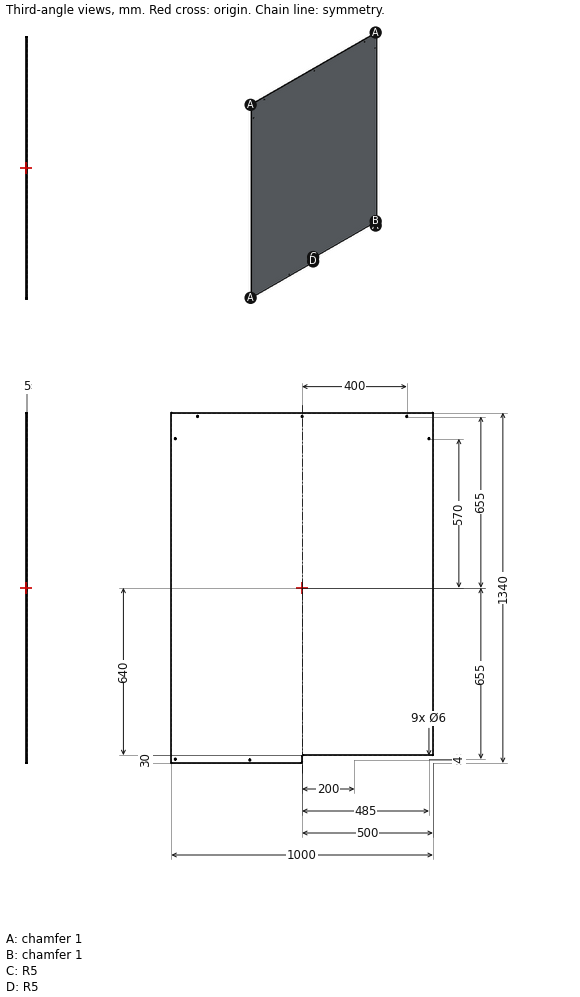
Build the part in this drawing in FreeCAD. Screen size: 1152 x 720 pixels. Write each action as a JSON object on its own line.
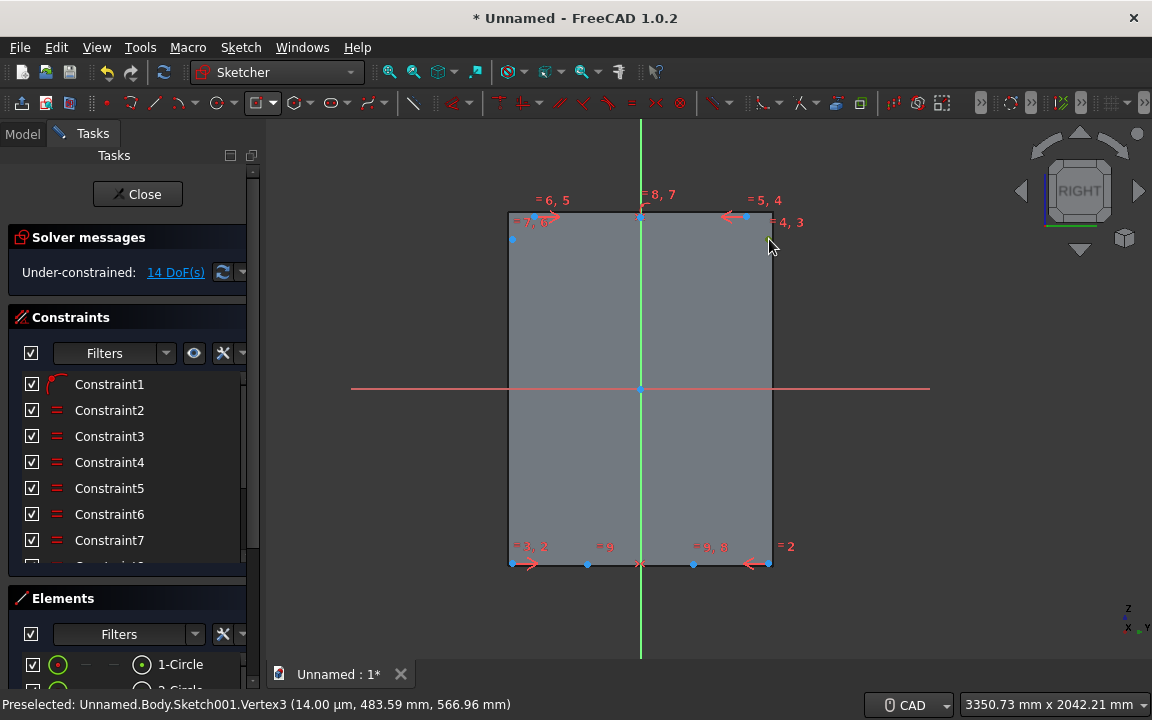
{"action": "left_click", "coordinate": [513, 239]}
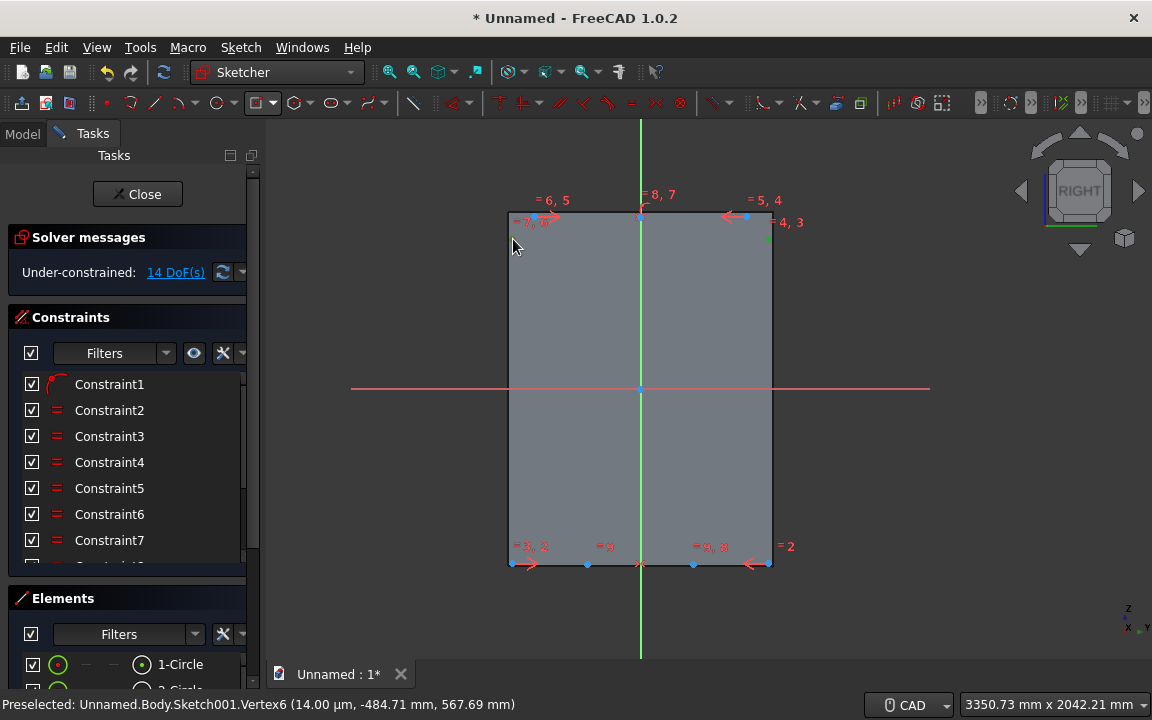
{"action": "left_click", "coordinate": [641, 596]}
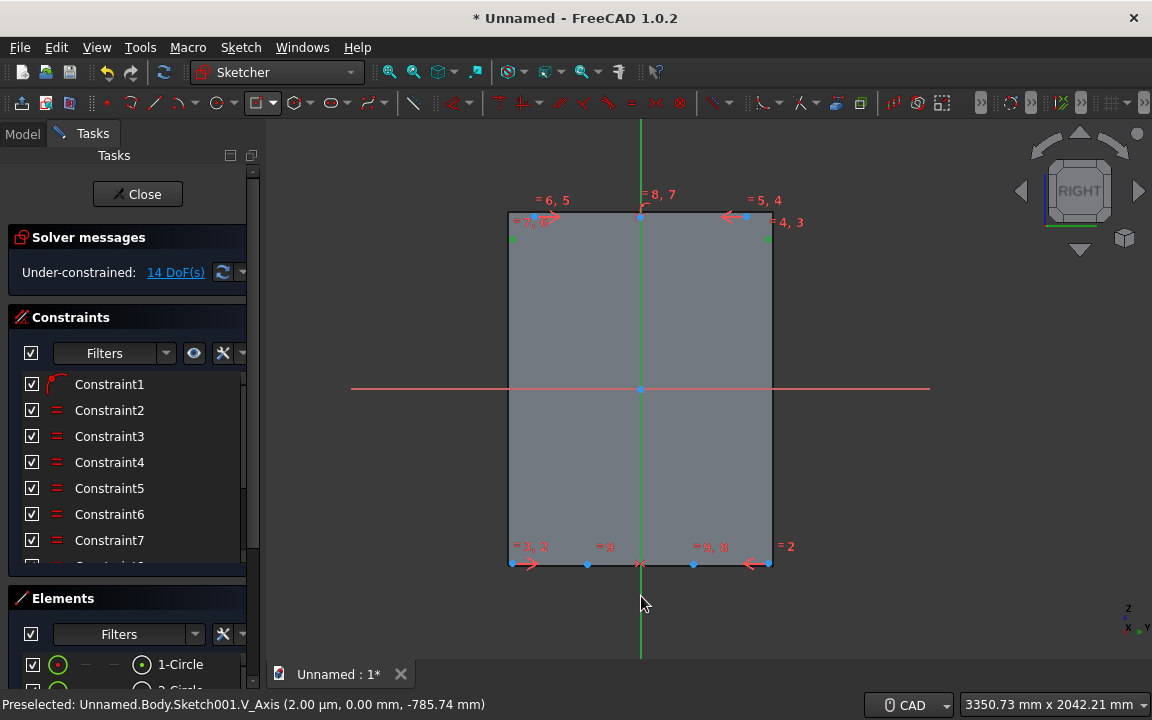
{"action": "left_click", "coordinate": [656, 104]}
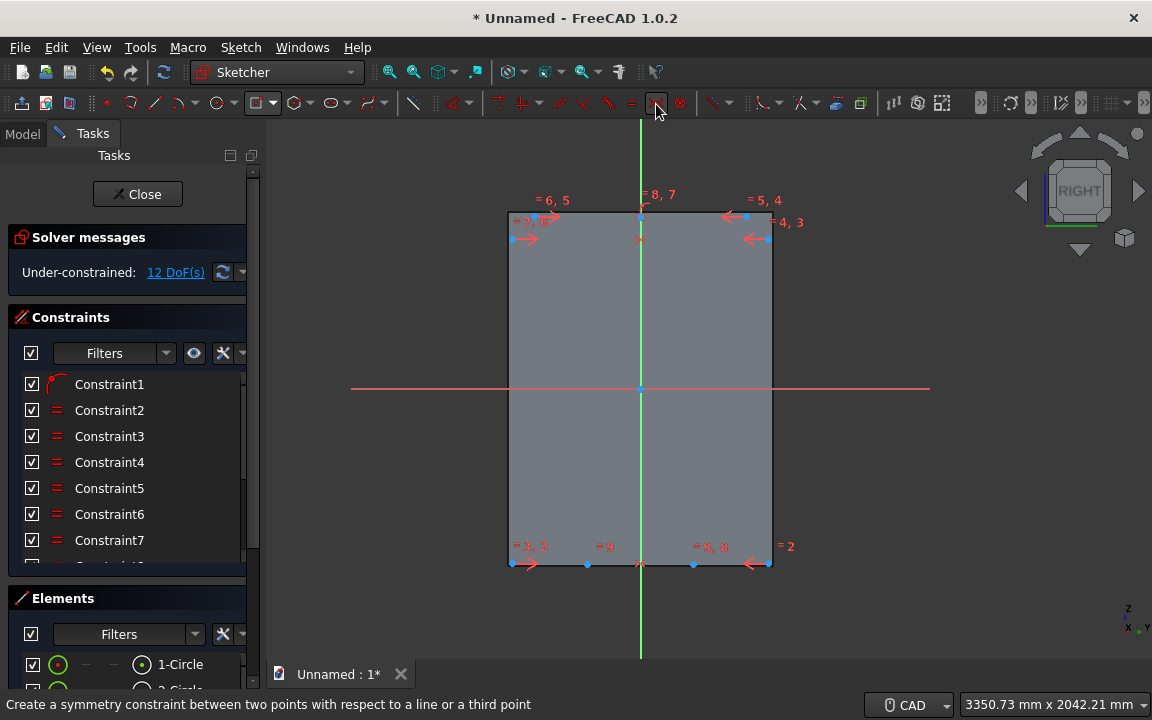
{"action": "left_click", "coordinate": [693, 564]}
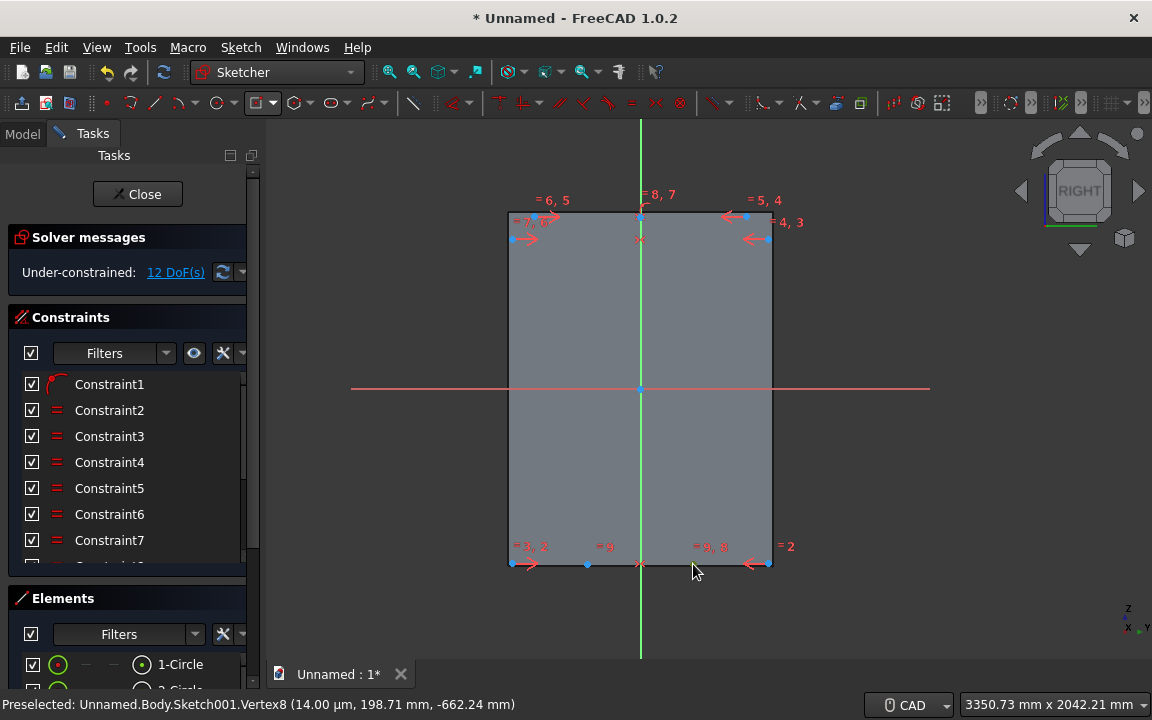
{"action": "left_click", "coordinate": [588, 564]}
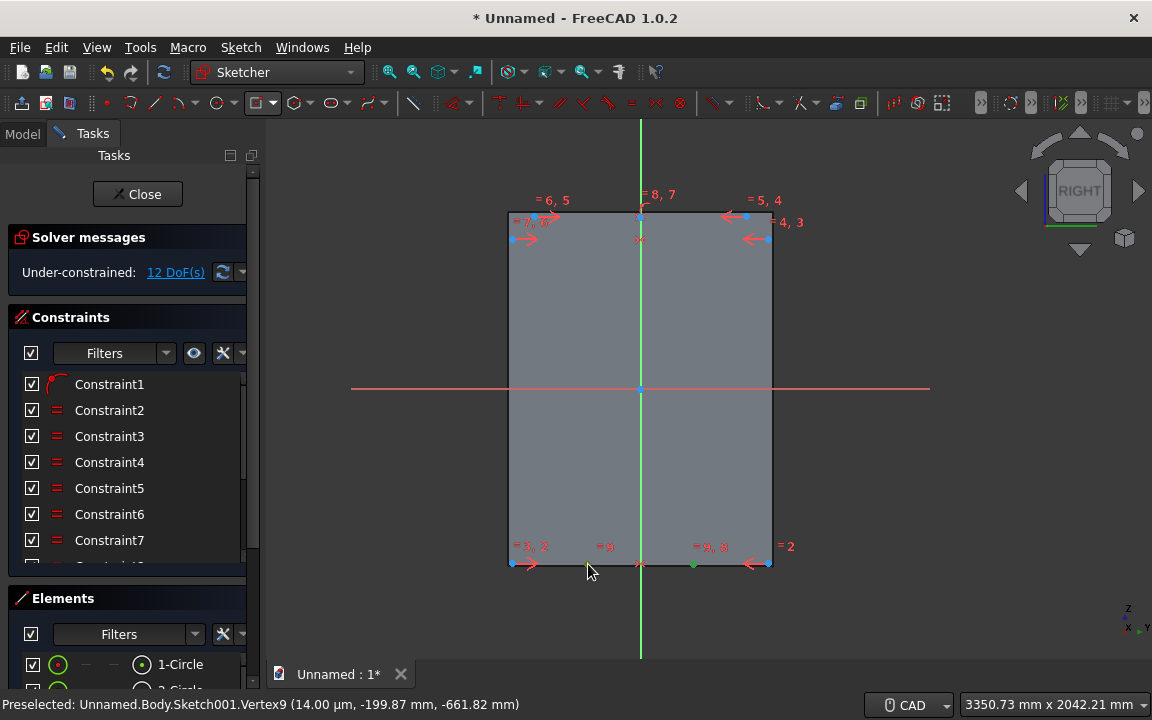
{"action": "left_click", "coordinate": [641, 596]}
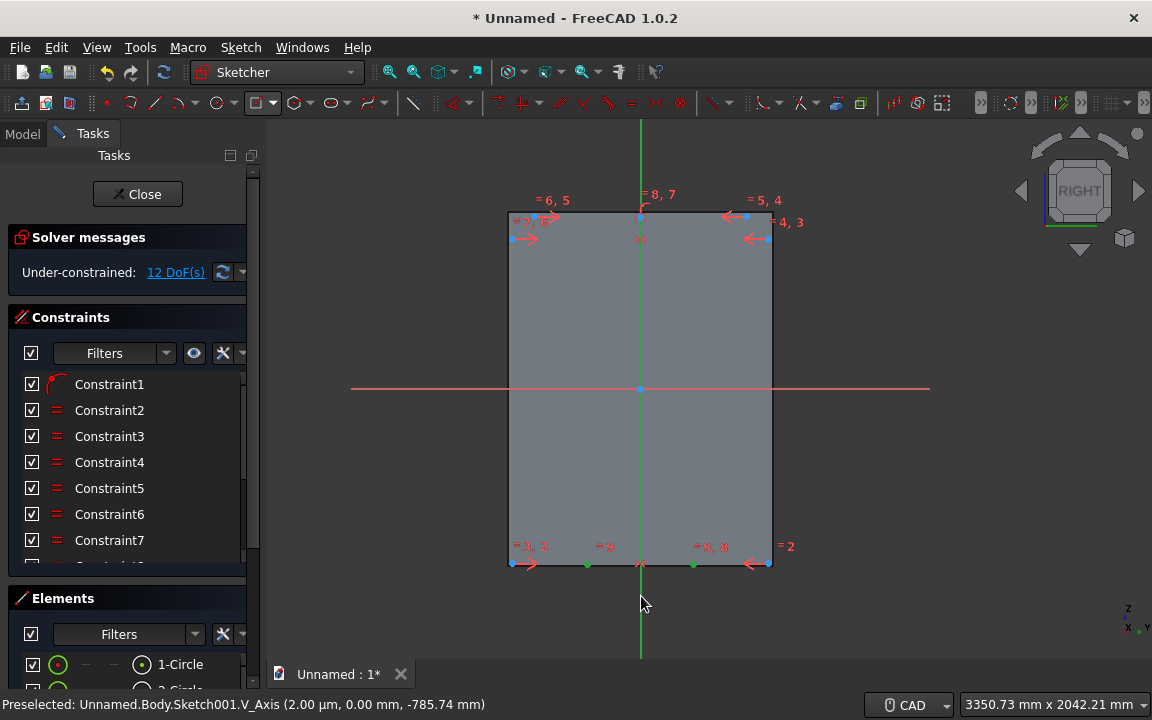
{"action": "left_click", "coordinate": [656, 104]}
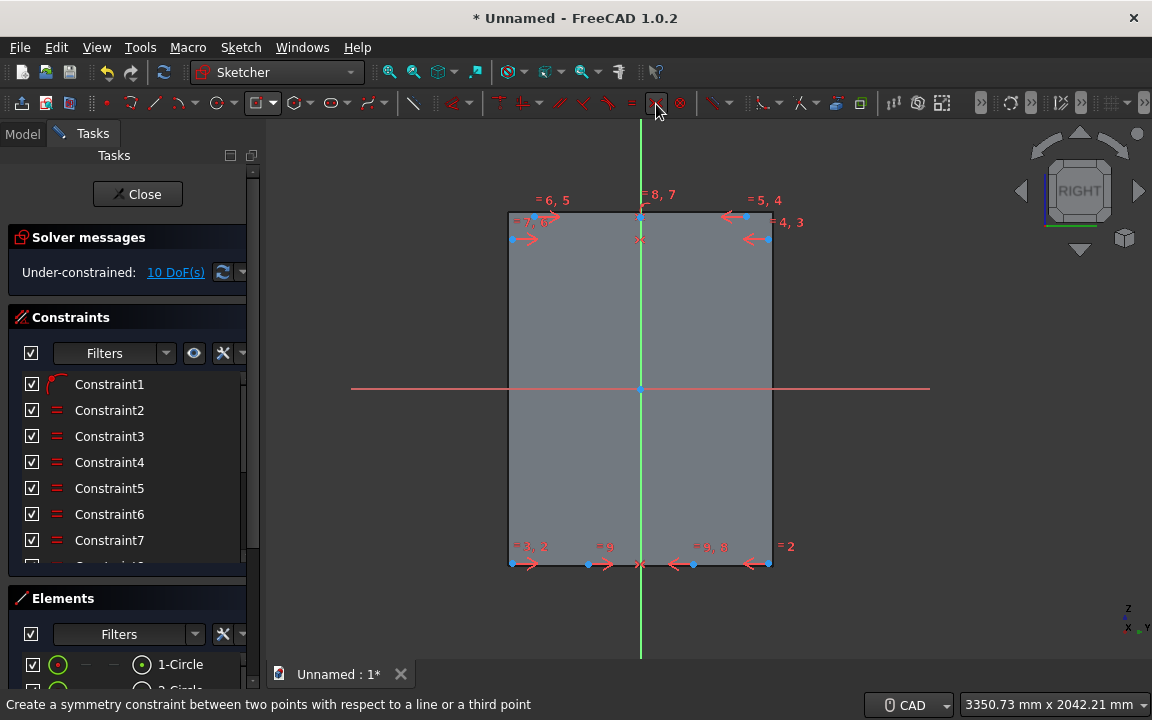
{"action": "left_click", "coordinate": [452, 104]}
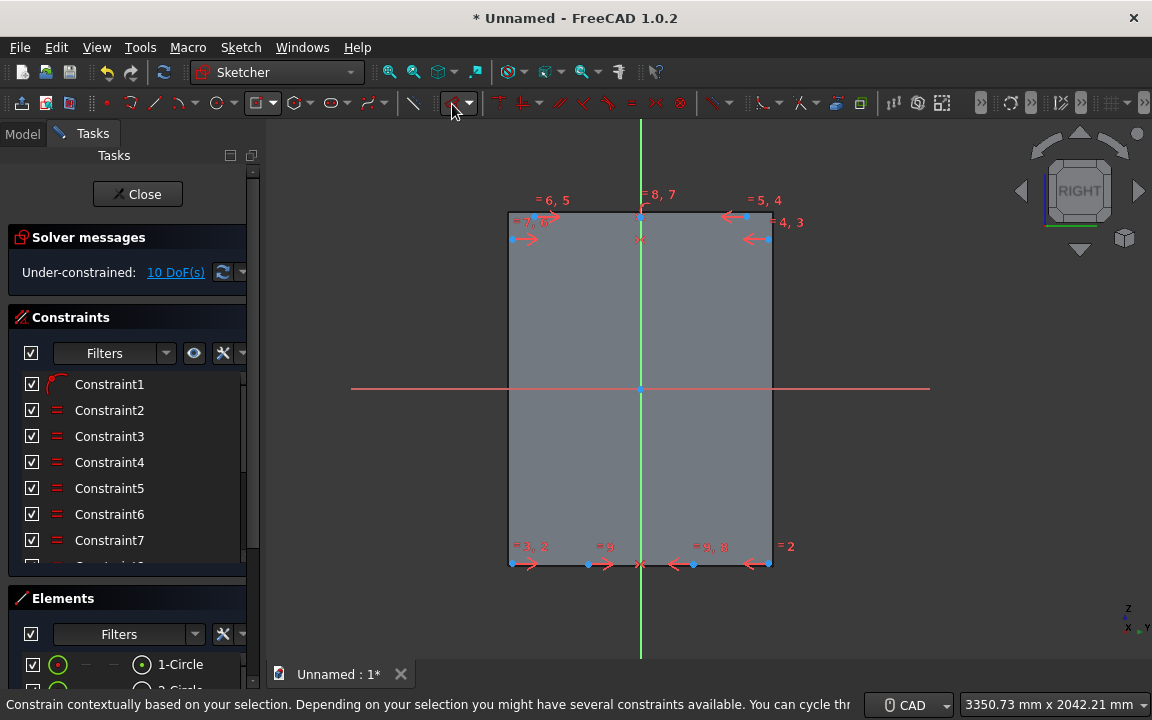
{"action": "scroll", "coordinate": [767, 562], "scroll_direction": "up", "scroll_amount": 17}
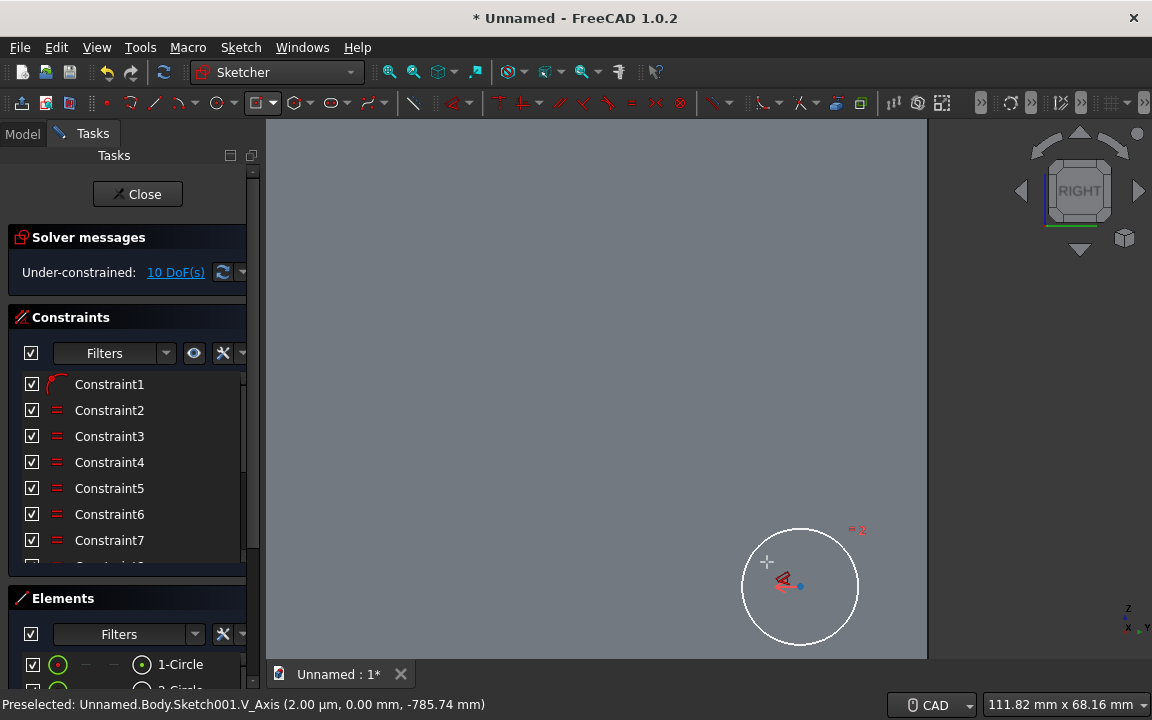
{"action": "left_click", "coordinate": [759, 546]}
{"action": "left_click", "coordinate": [736, 523]}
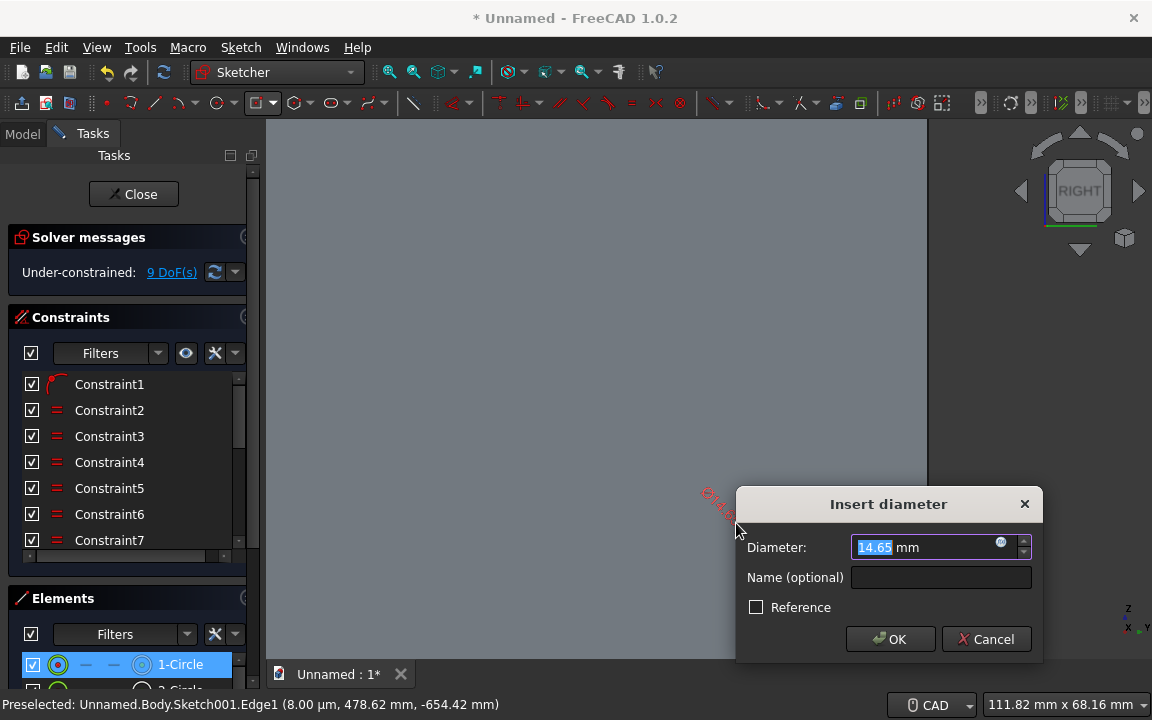
{"action": "type", "text": "6"}
{"action": "key", "text": "Return"}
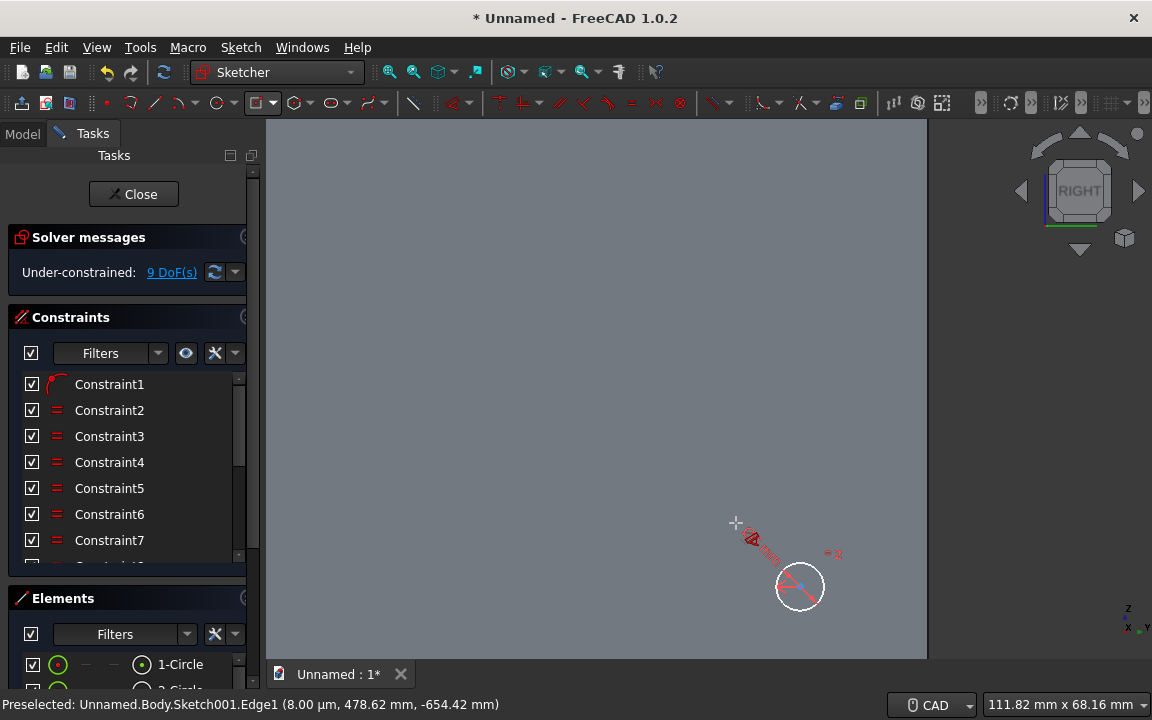
{"action": "scroll", "coordinate": [800, 587], "scroll_direction": "up", "scroll_amount": 2}